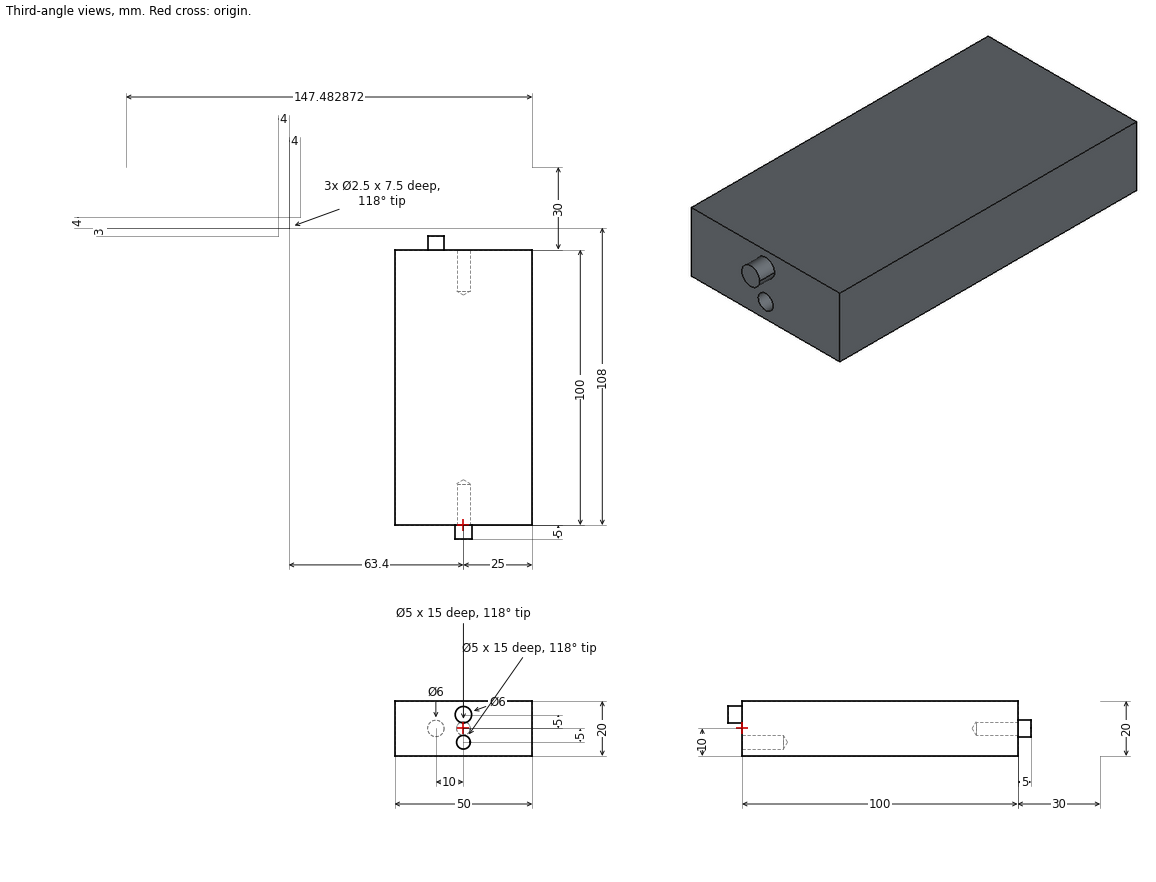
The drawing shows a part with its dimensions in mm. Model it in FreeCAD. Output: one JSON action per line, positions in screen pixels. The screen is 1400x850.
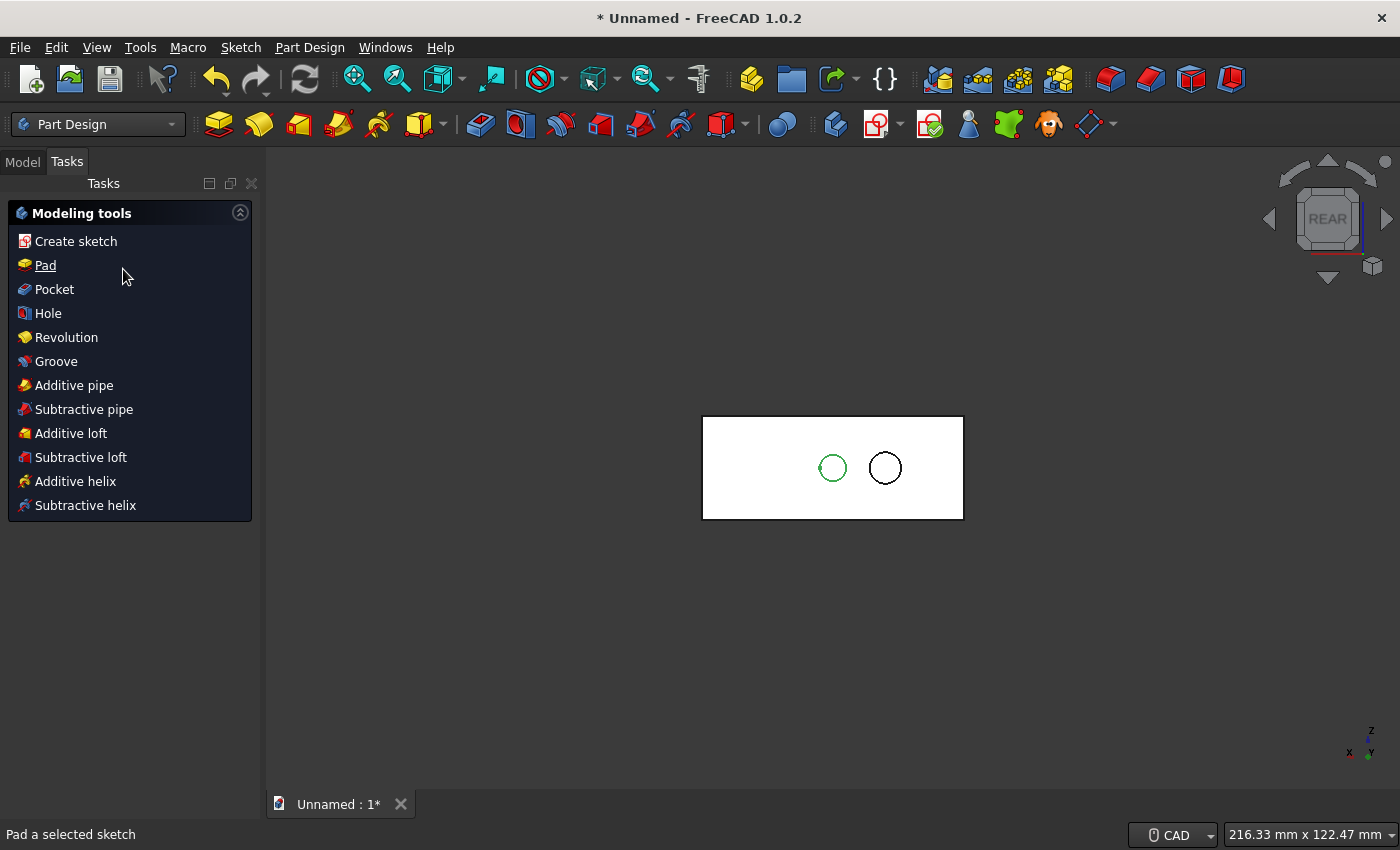
{"action": "left_click", "coordinate": [522, 124]}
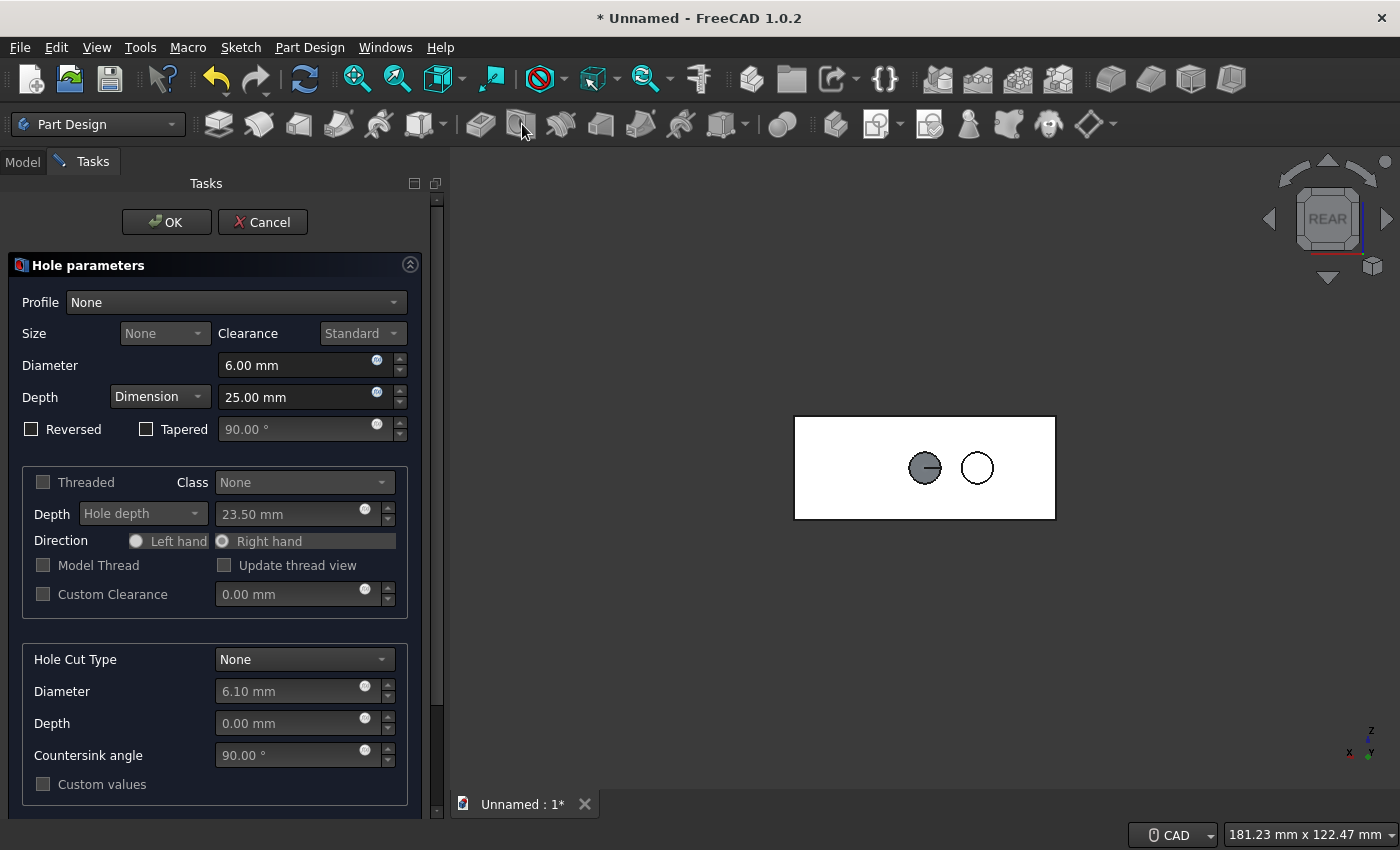
{"action": "triple_click", "coordinate": [305, 365]}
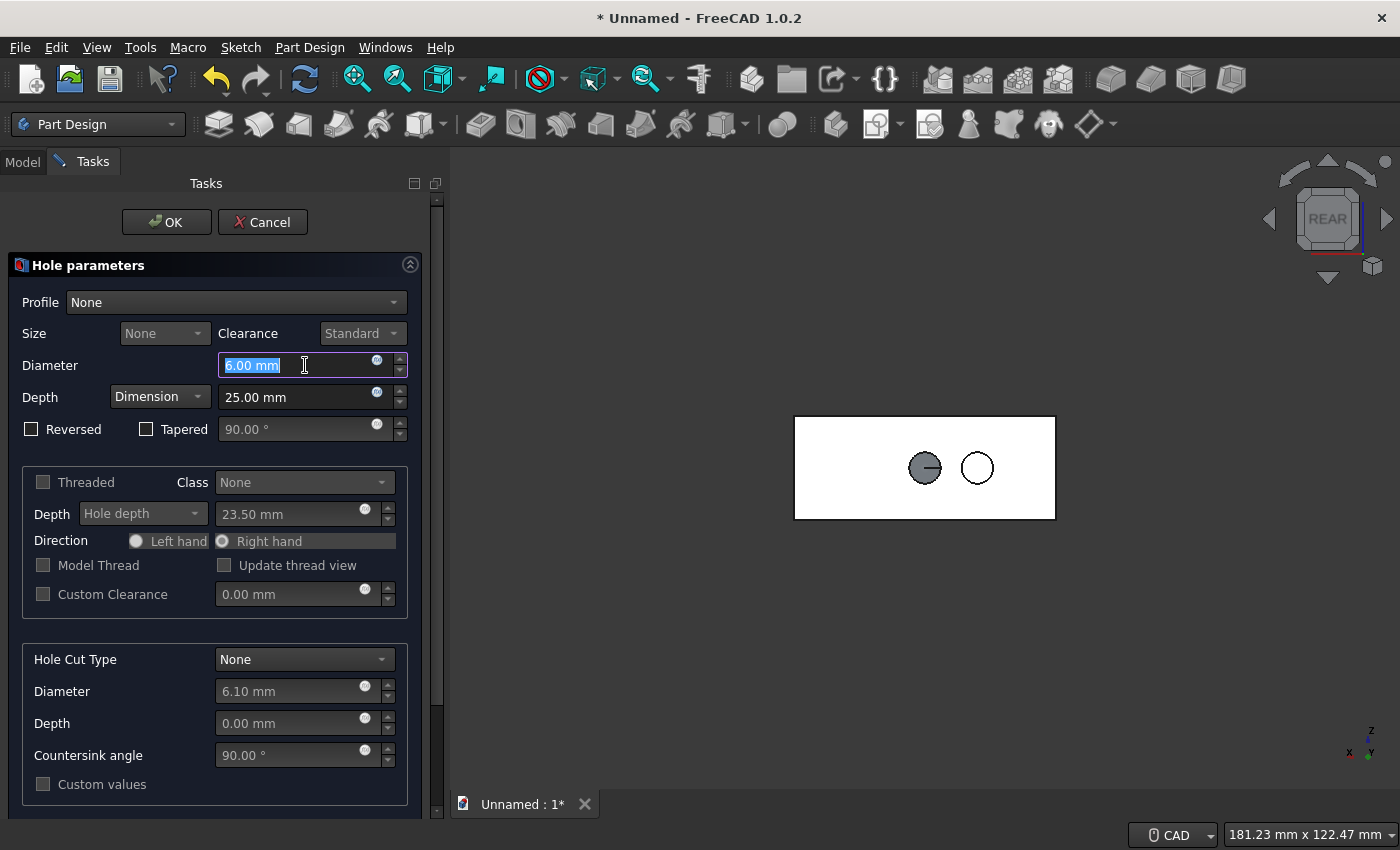
{"action": "type", "text": "5"}
{"action": "key", "text": "Tab"}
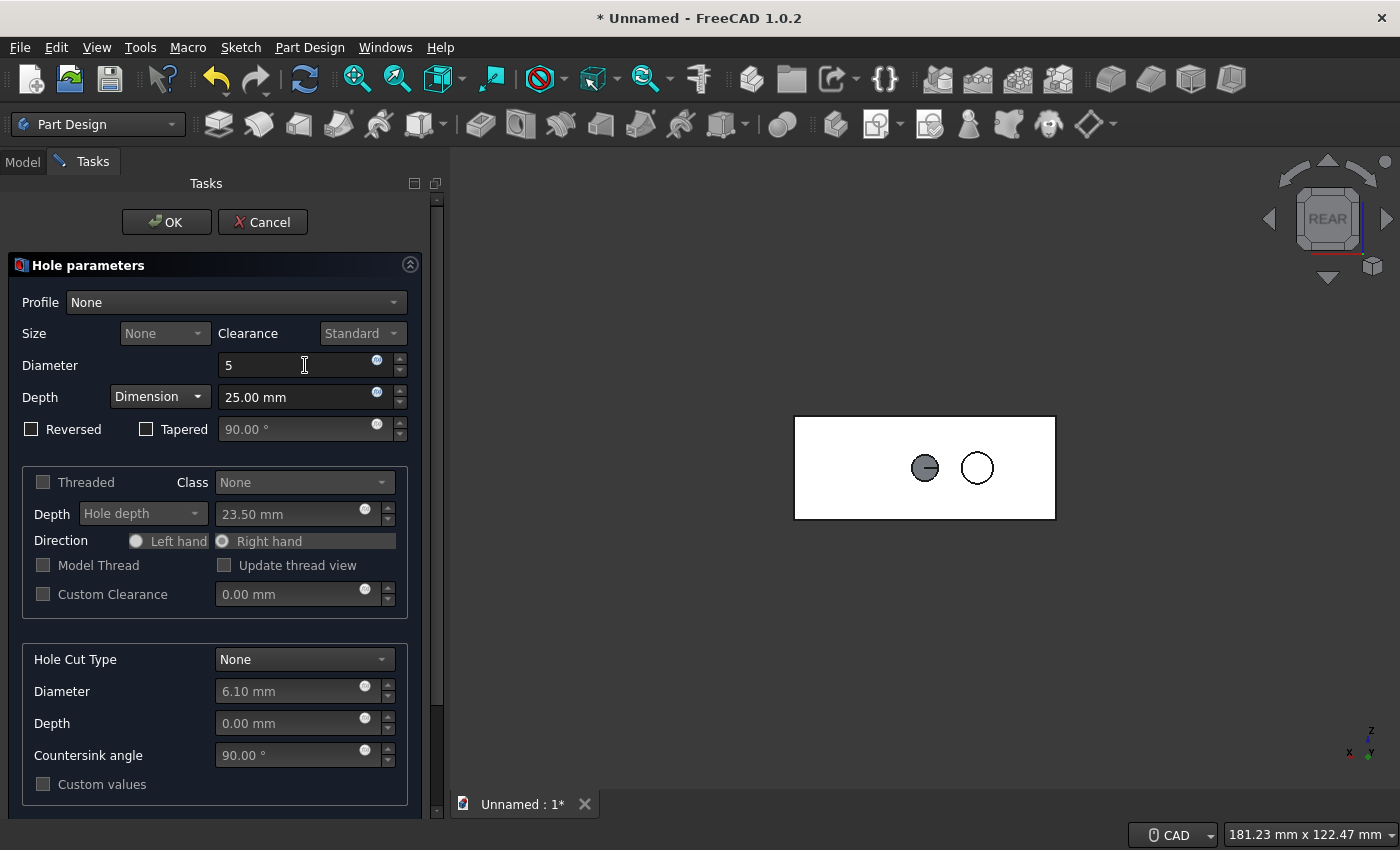
{"action": "triple_click", "coordinate": [305, 397]}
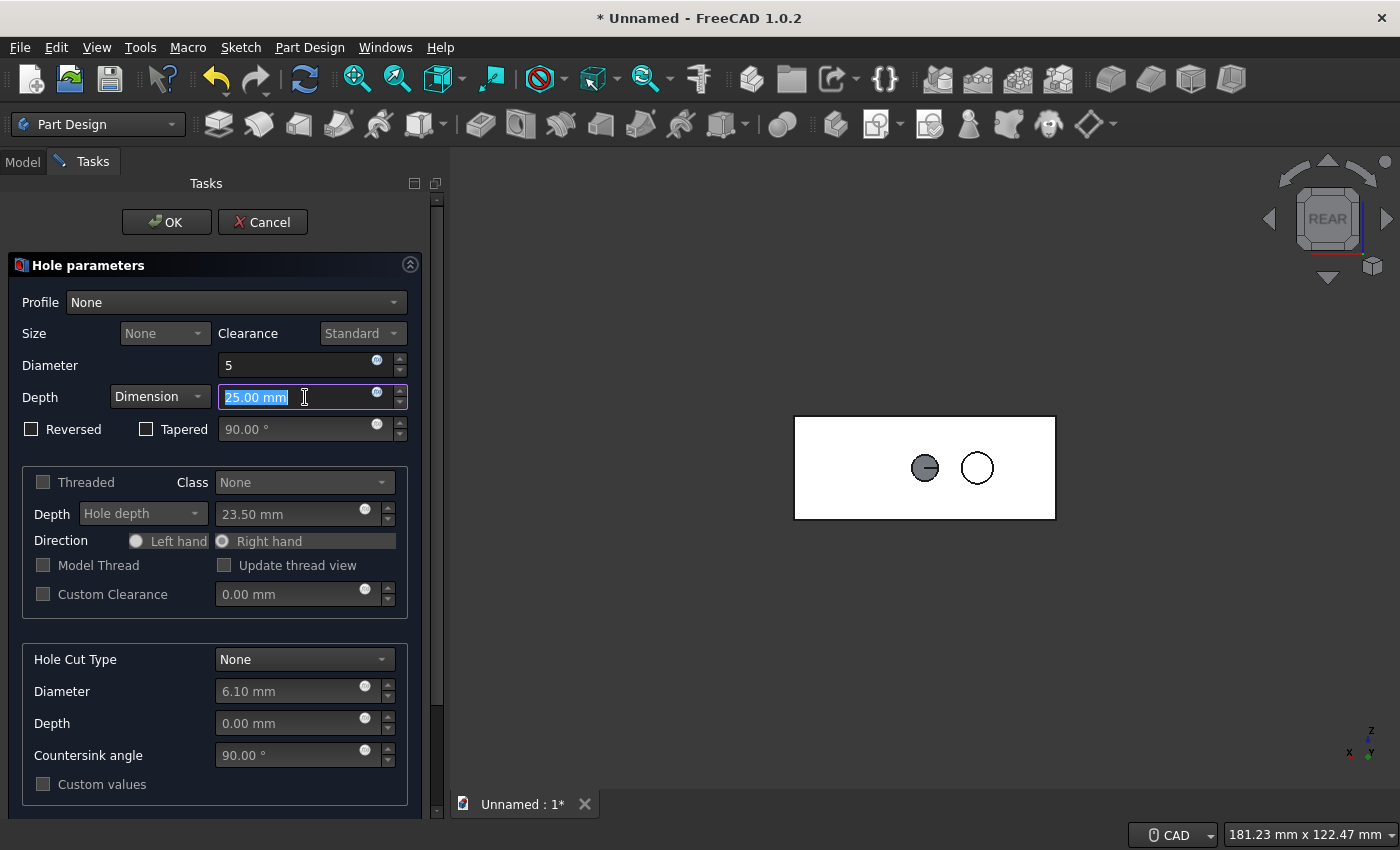
{"action": "type", "text": "15"}
{"action": "key", "text": "Tab"}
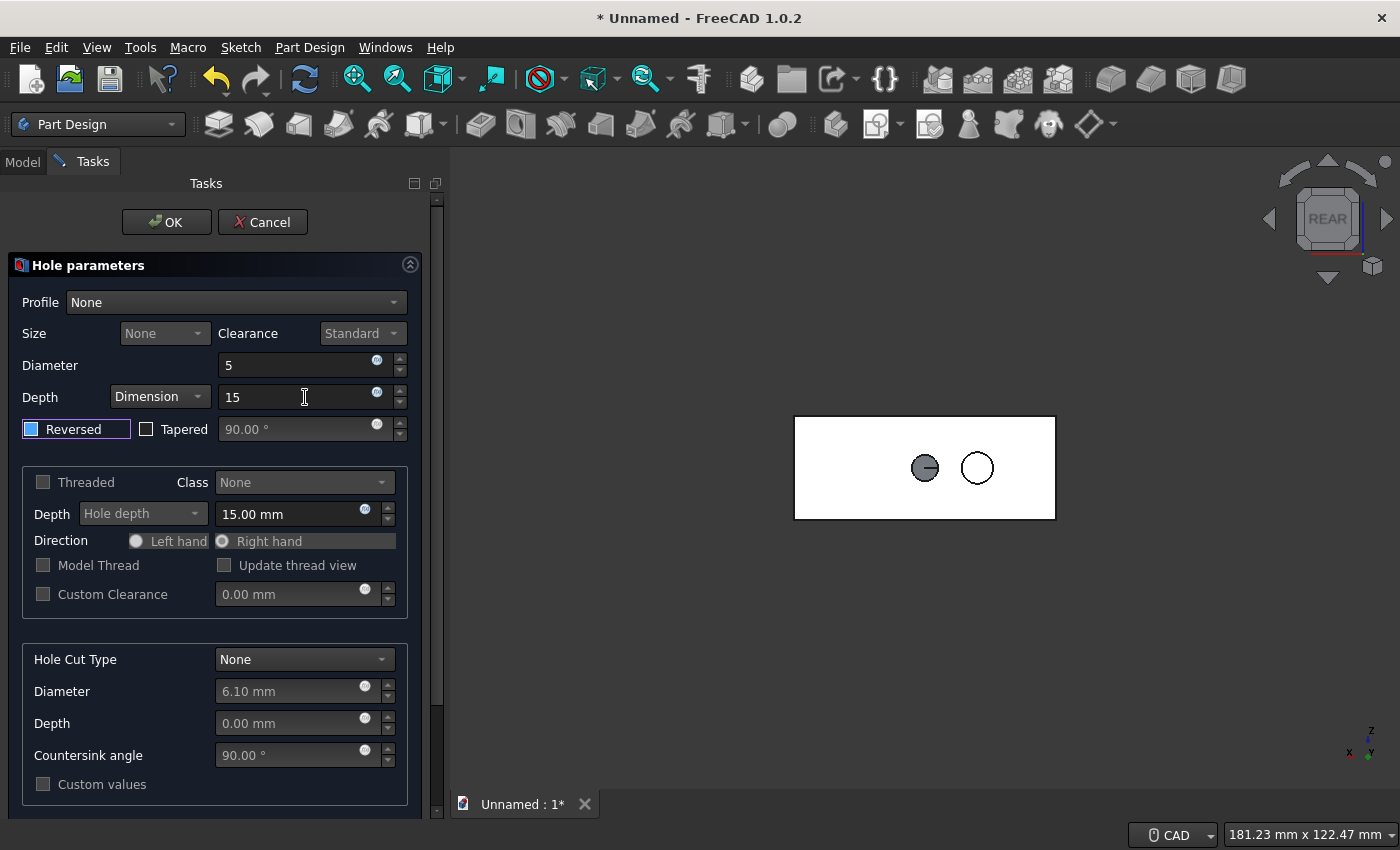
{"action": "left_click", "coordinate": [167, 222]}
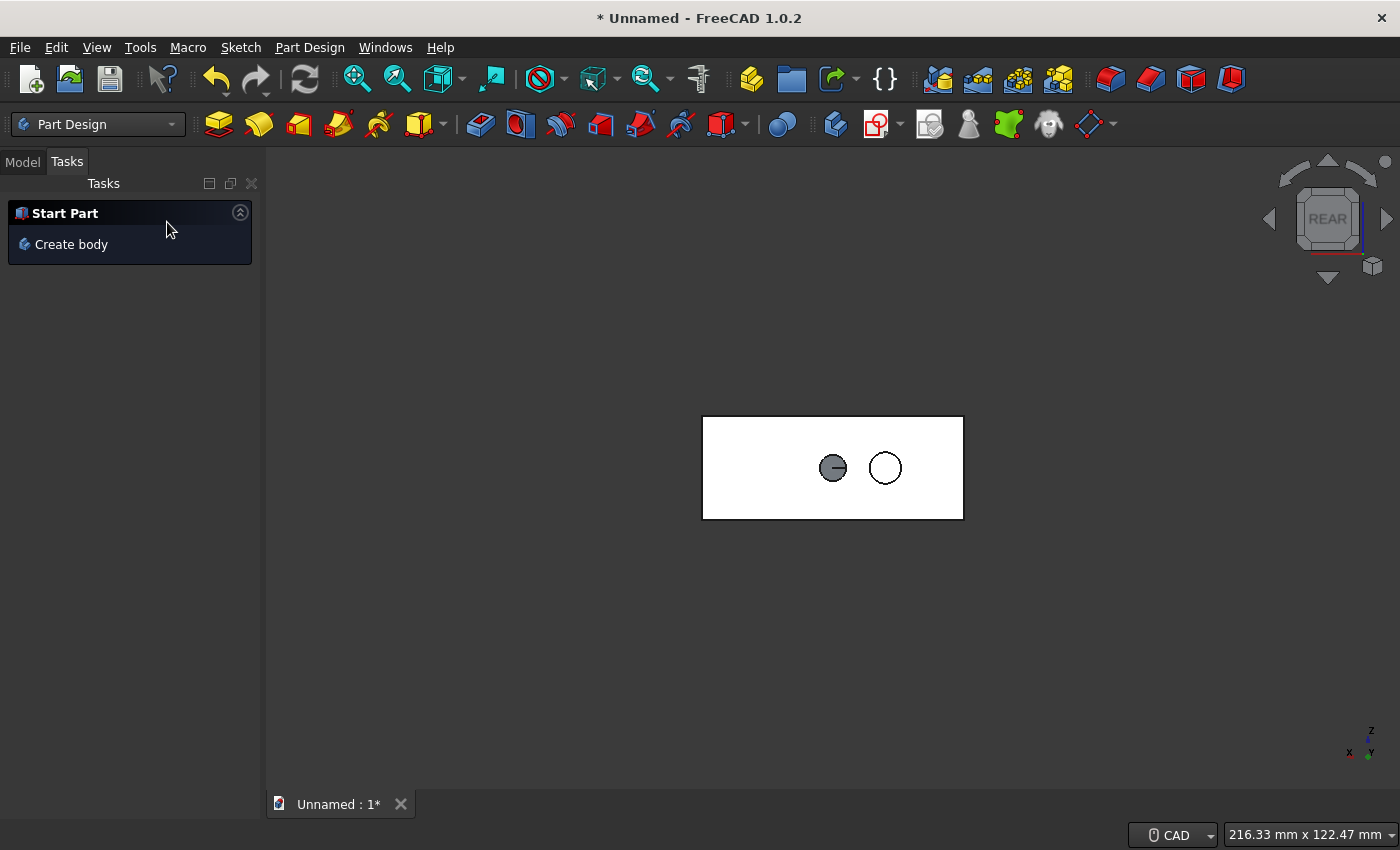
{"action": "key", "text": "0"}